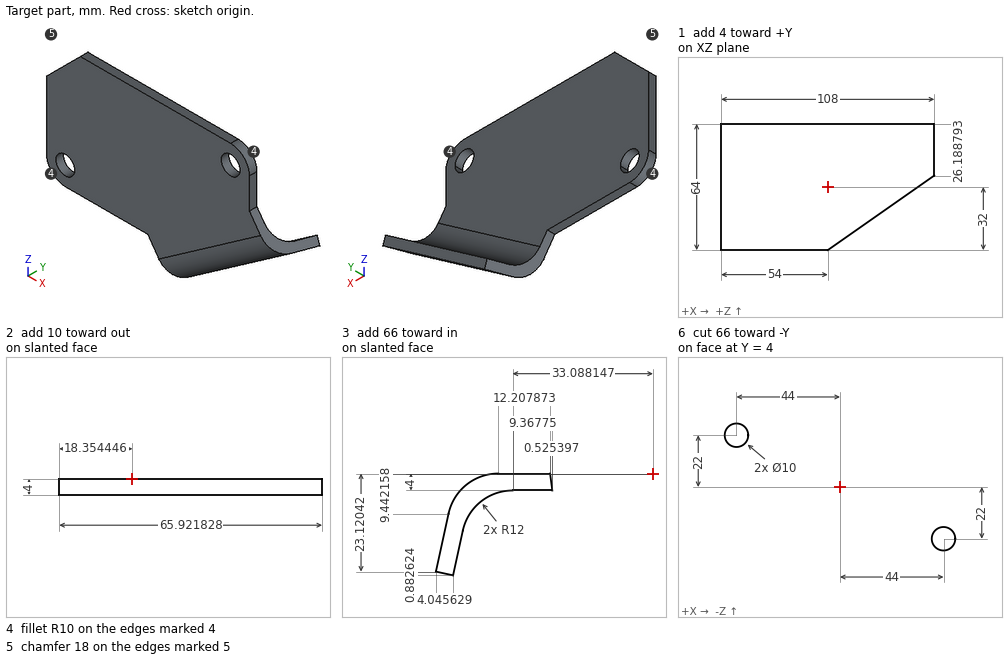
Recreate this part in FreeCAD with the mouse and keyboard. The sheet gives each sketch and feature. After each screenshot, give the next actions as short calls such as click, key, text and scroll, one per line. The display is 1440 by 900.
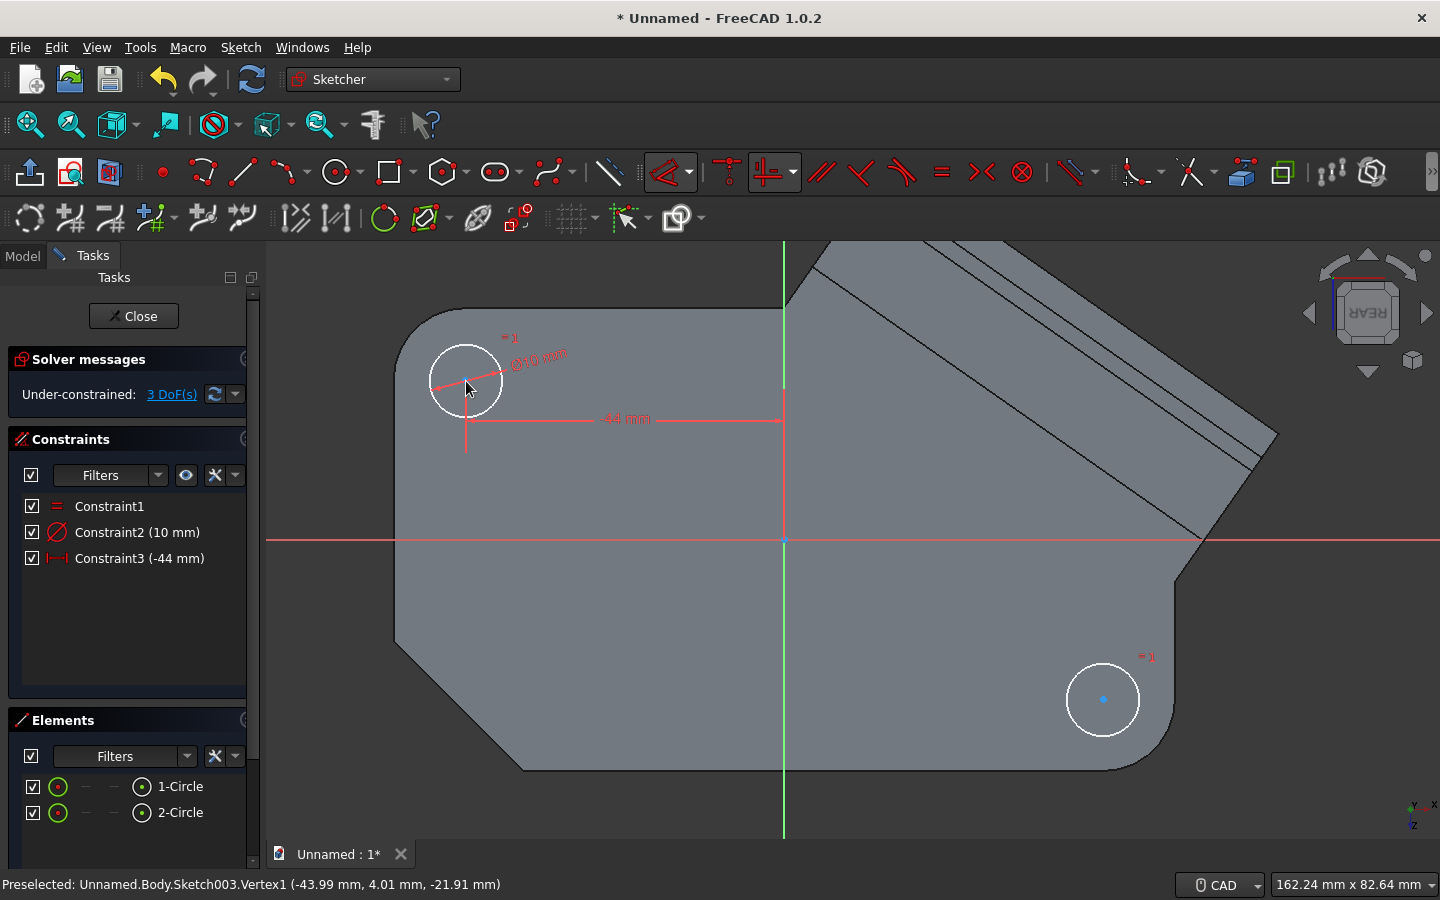
click(466, 381)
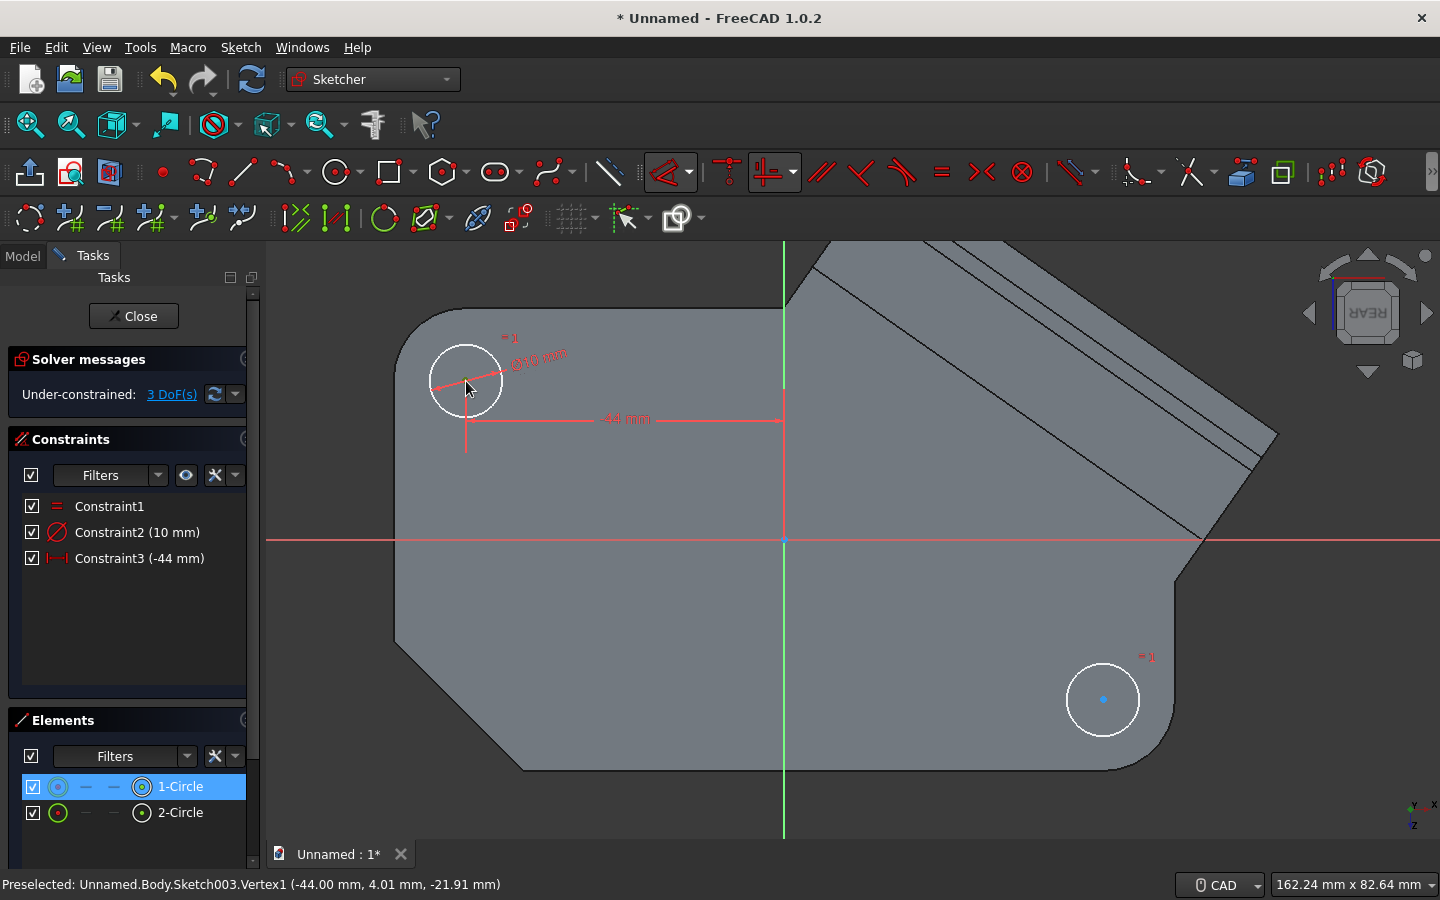
click(692, 172)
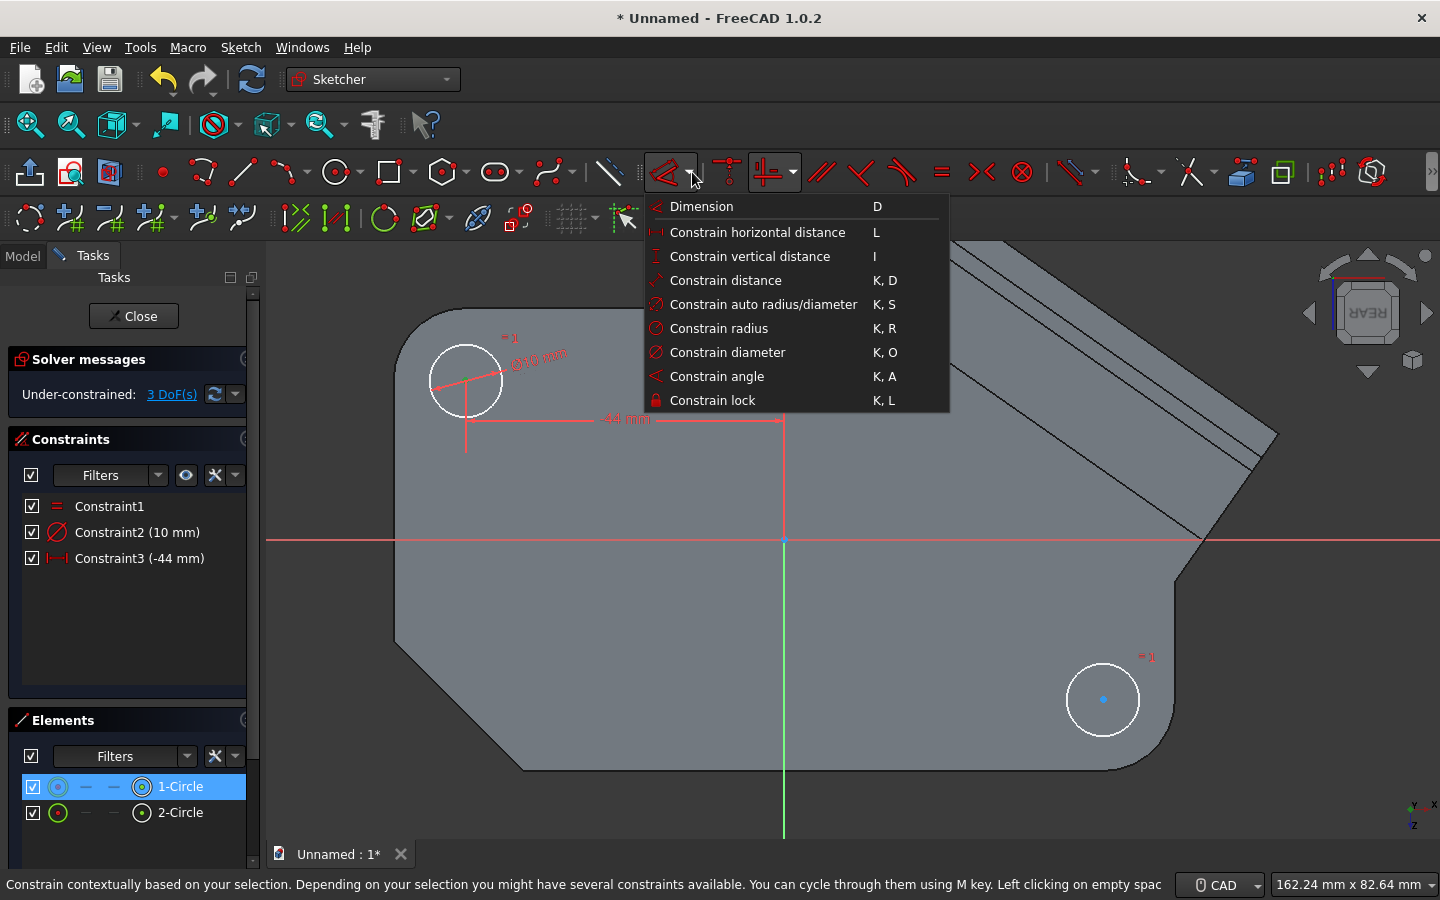
click(797, 256)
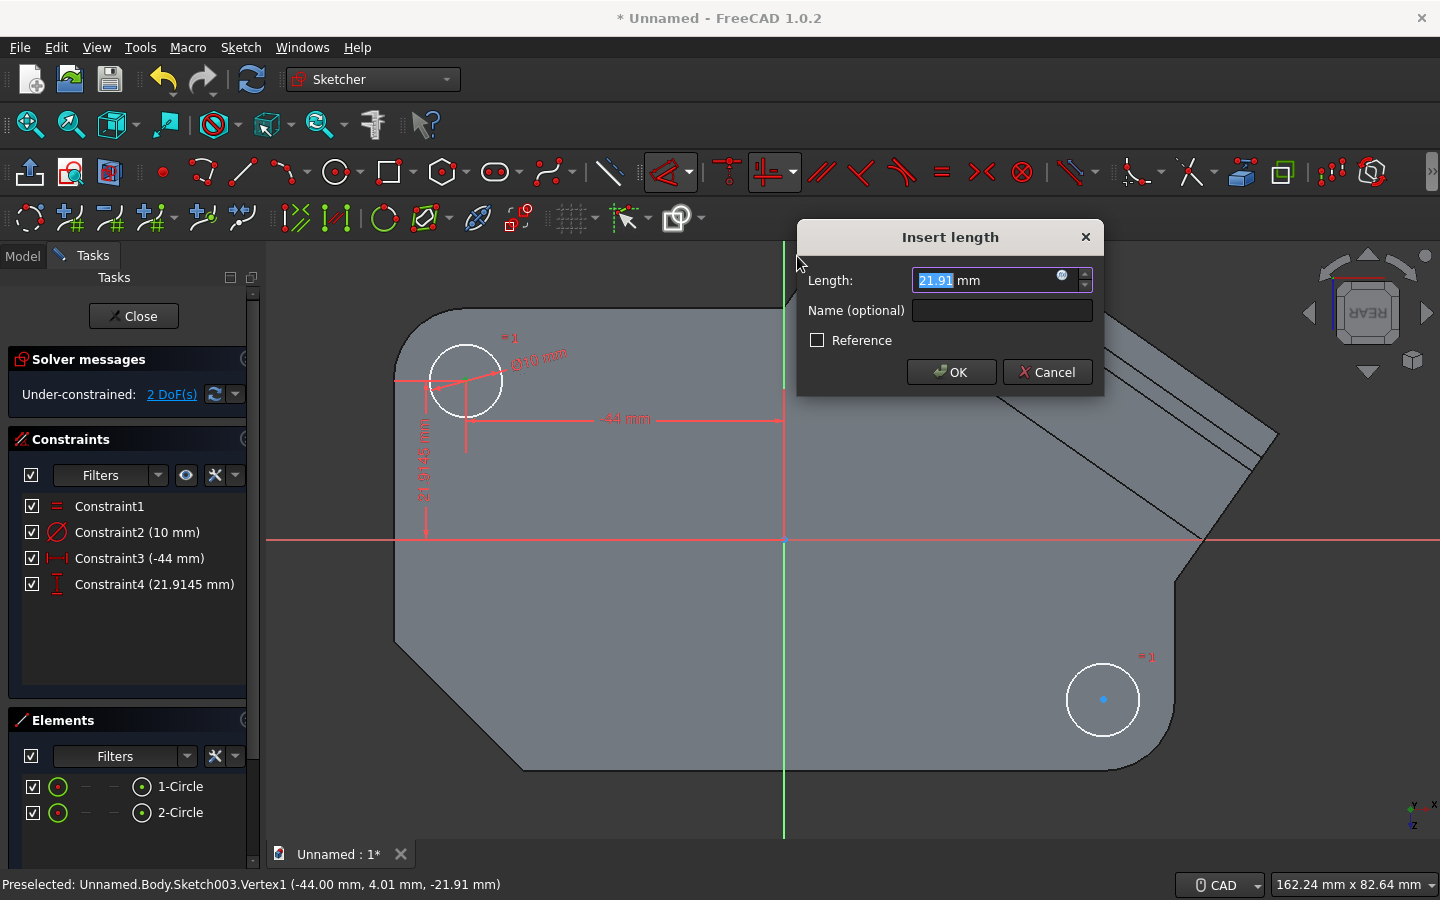
text(22)
key(Return)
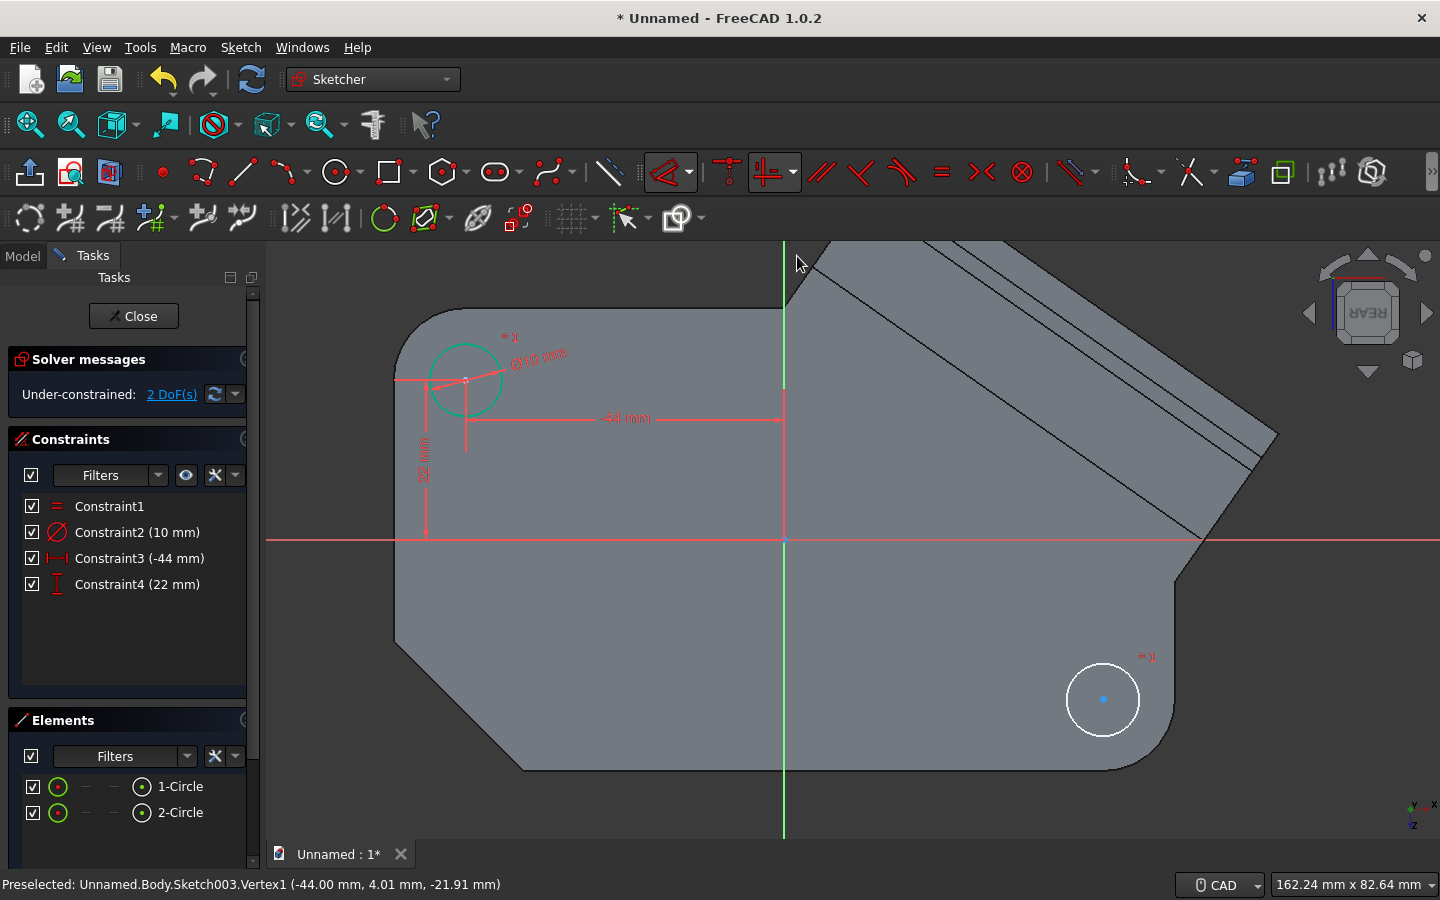
click(1103, 700)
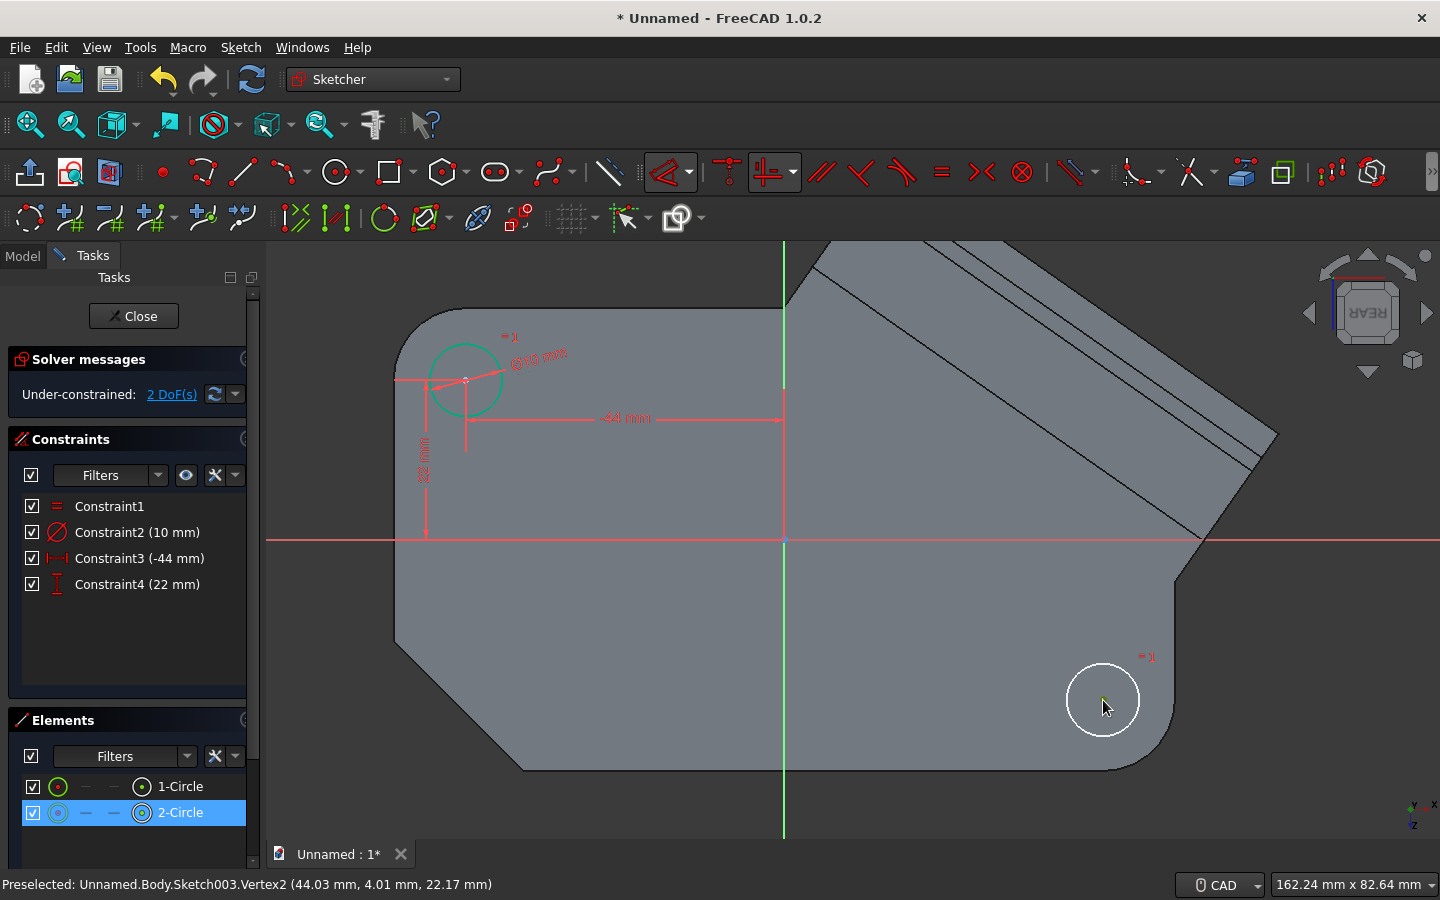
key(l)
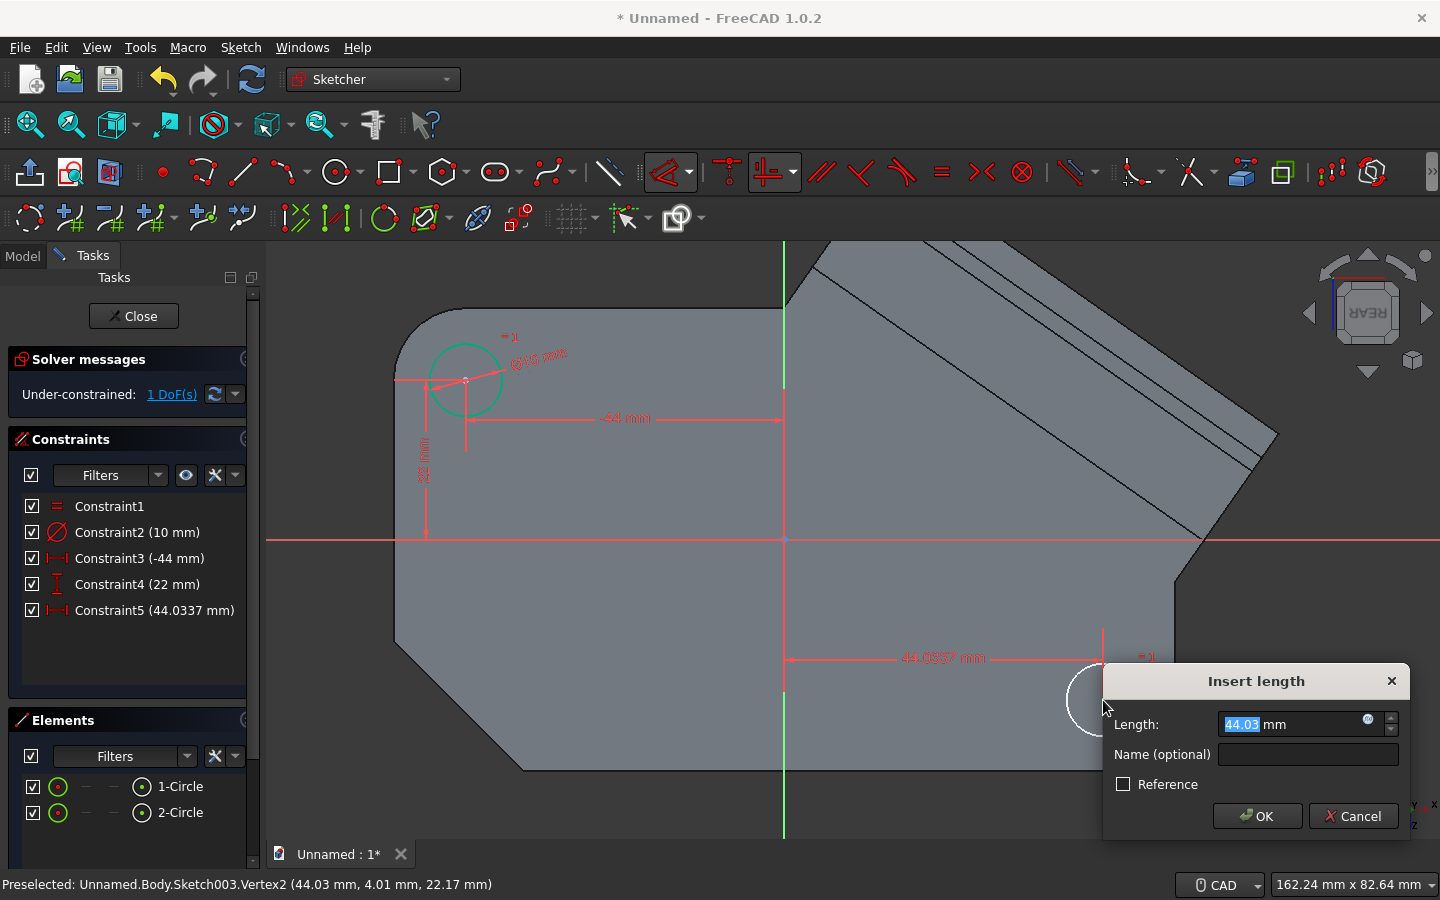
text(44)
key(Return)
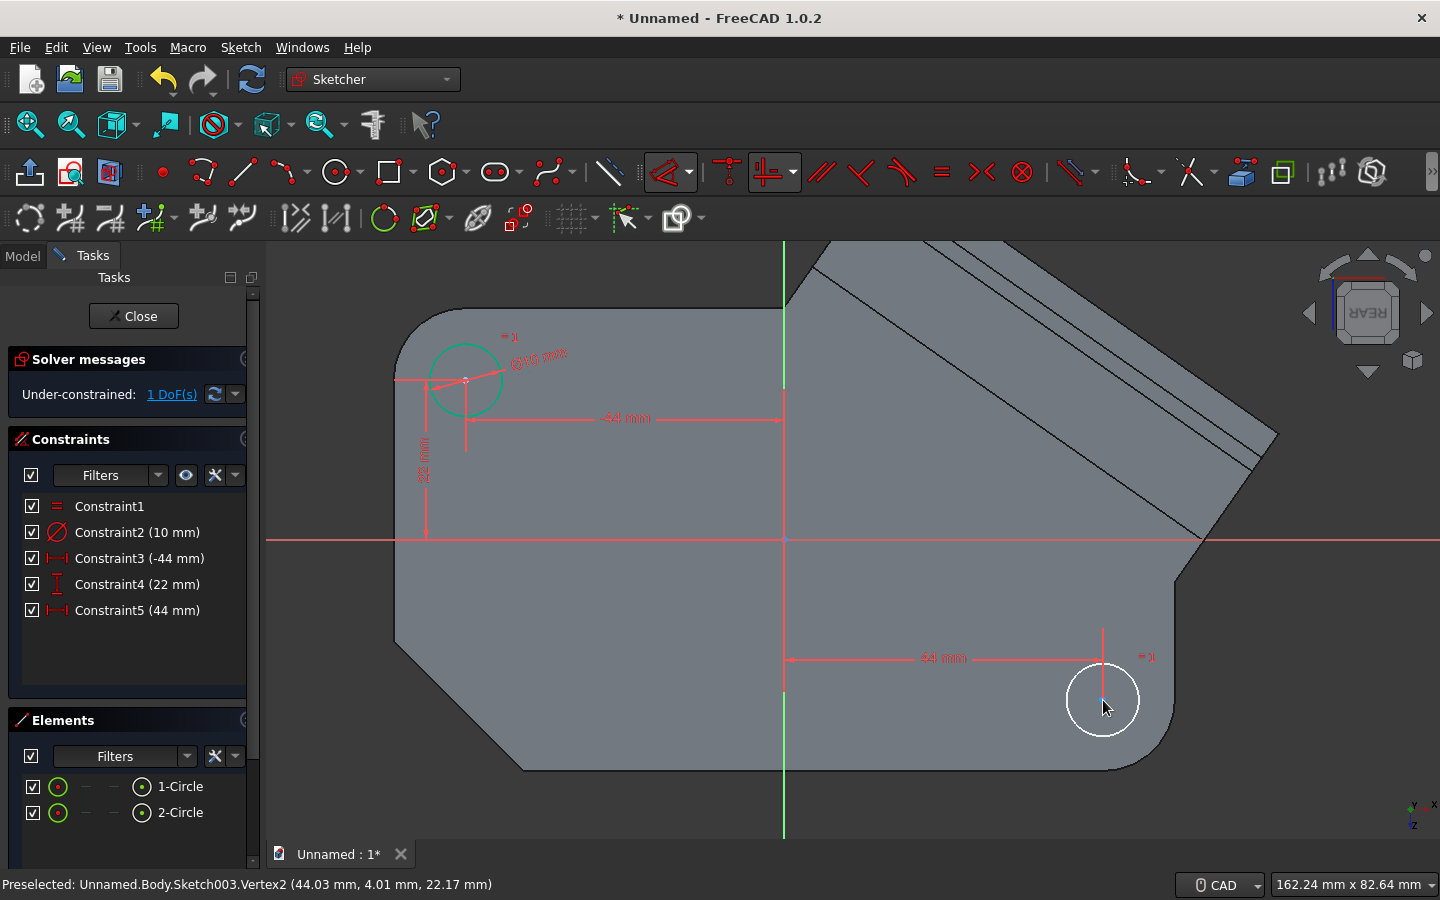
click(1103, 700)